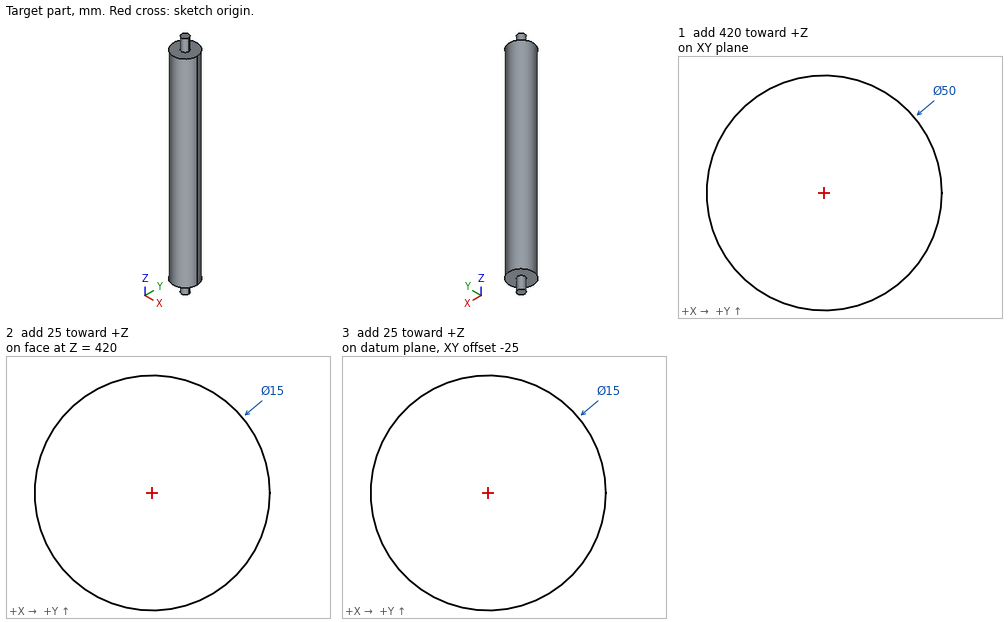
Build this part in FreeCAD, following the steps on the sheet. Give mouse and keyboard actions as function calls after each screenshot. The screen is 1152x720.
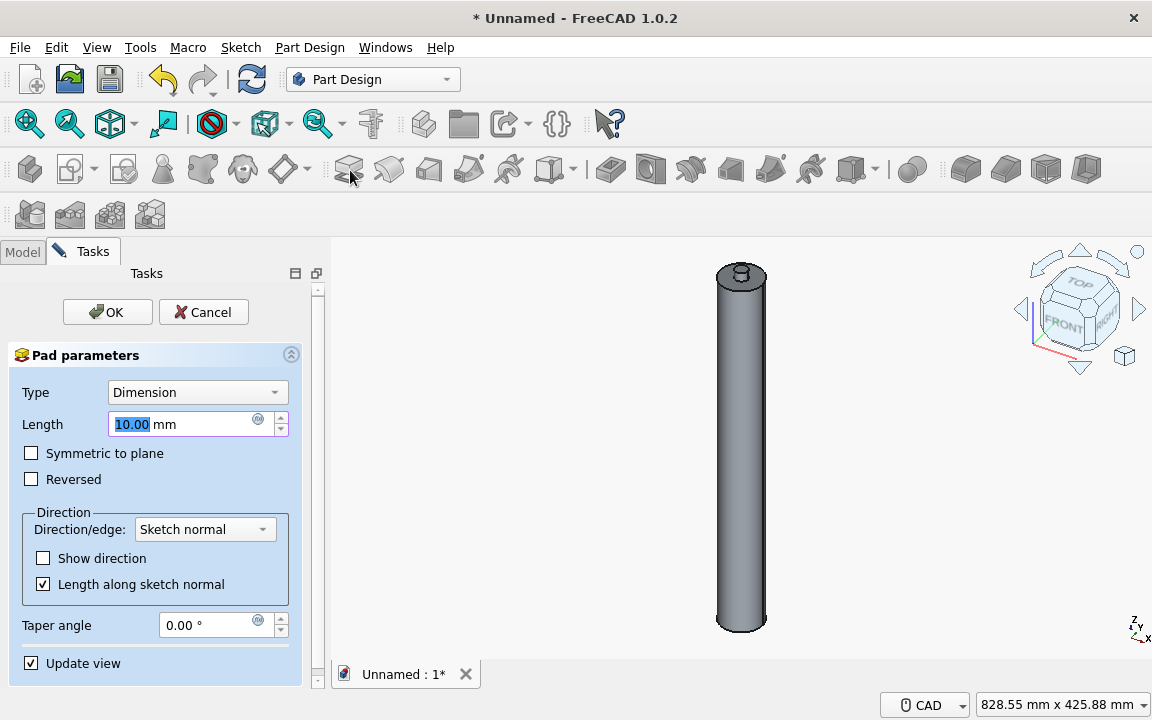
text(25)
key(Tab)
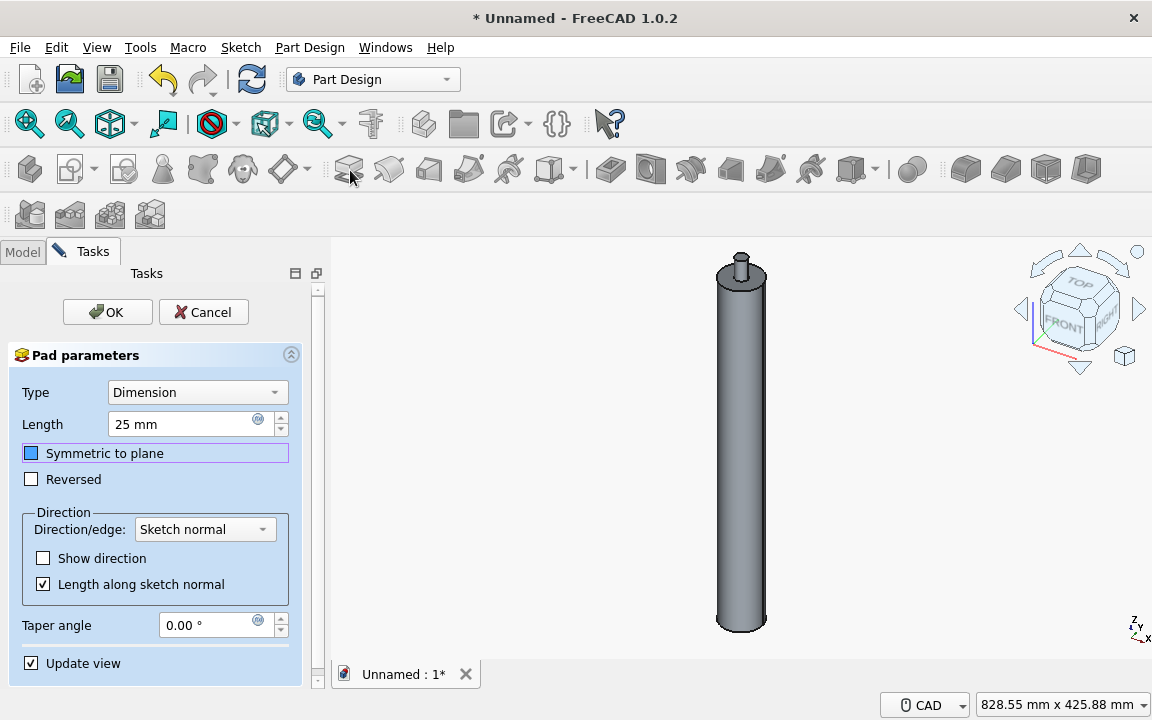
click(108, 312)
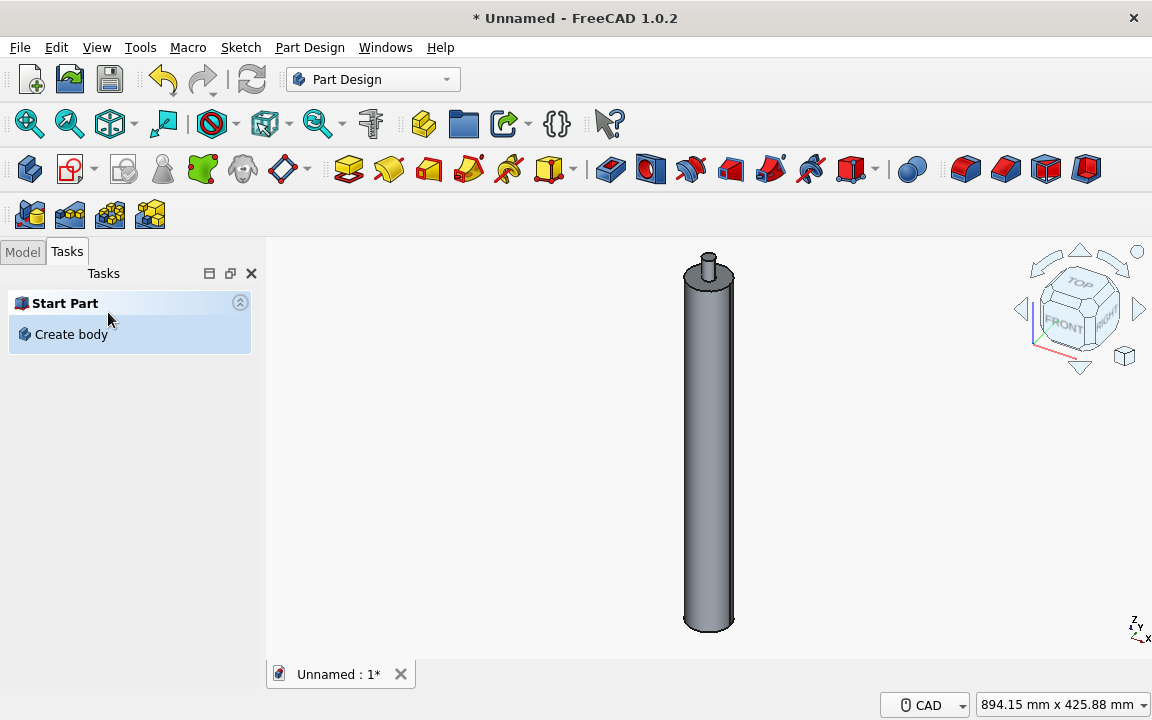
click(23, 251)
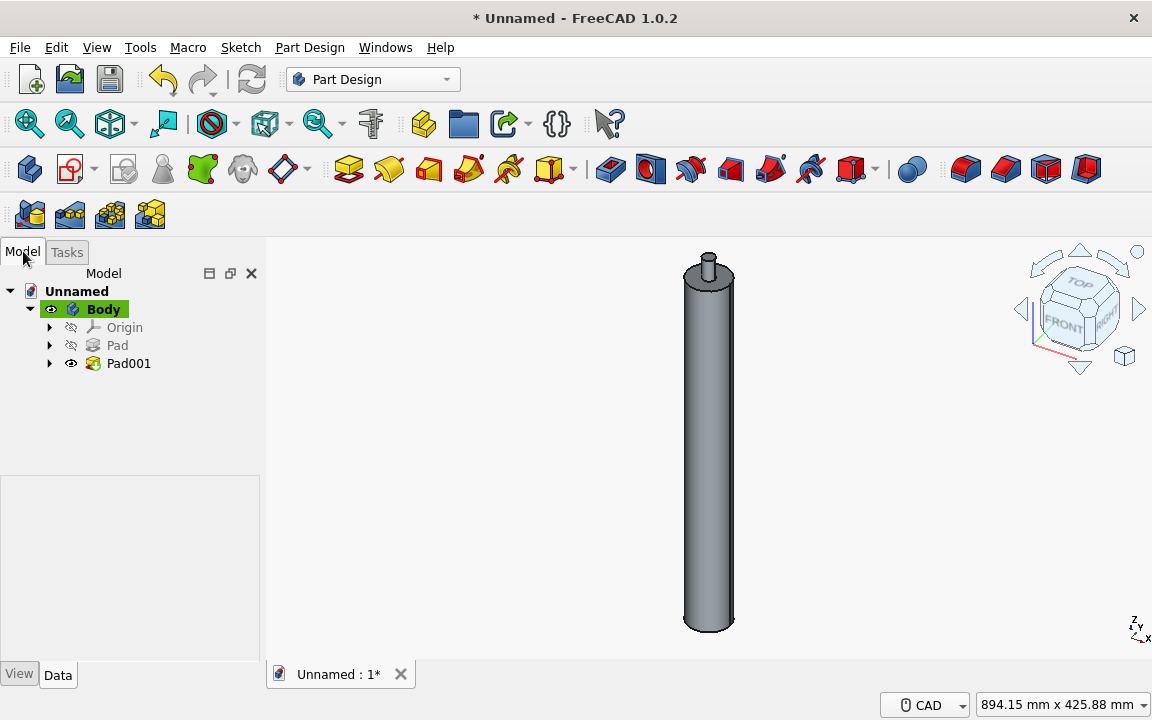
click(50, 327)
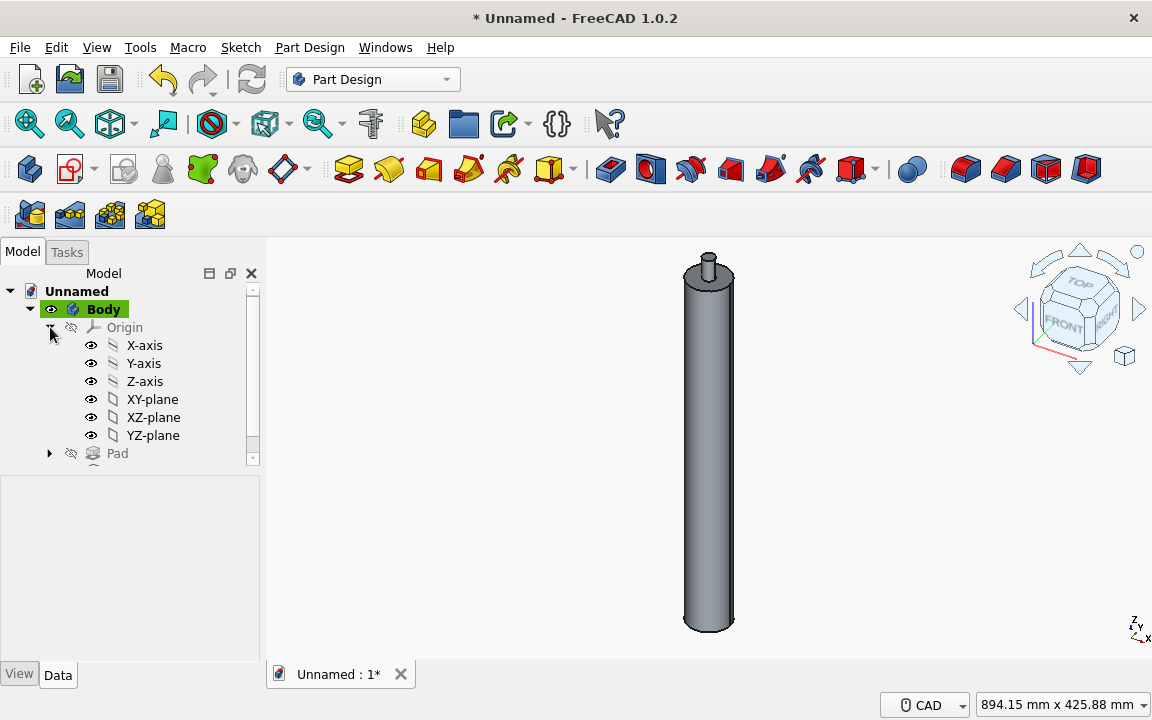
click(136, 399)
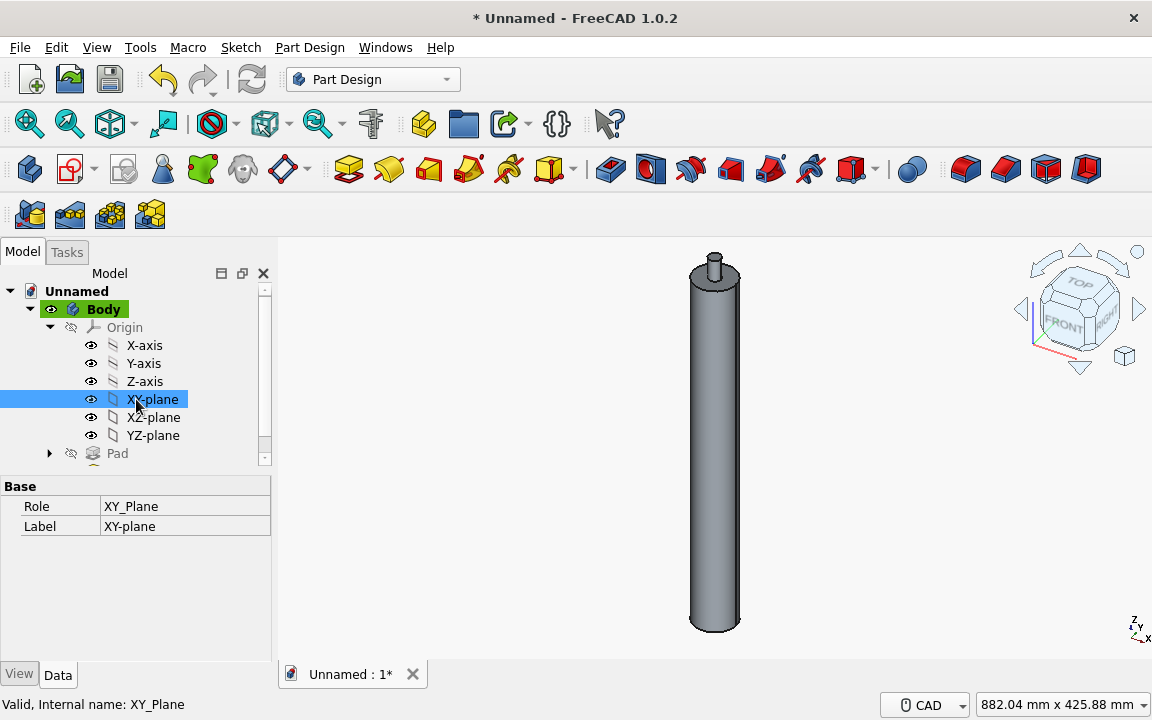
click(284, 170)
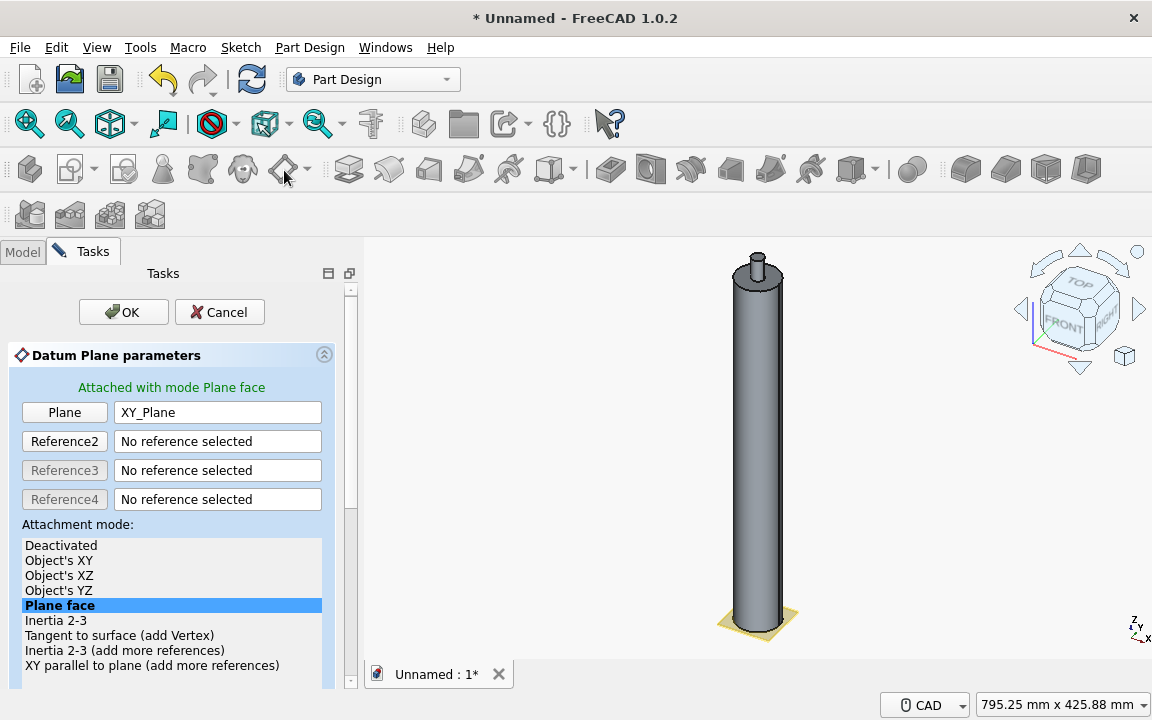
scroll(351, 486, down, 4)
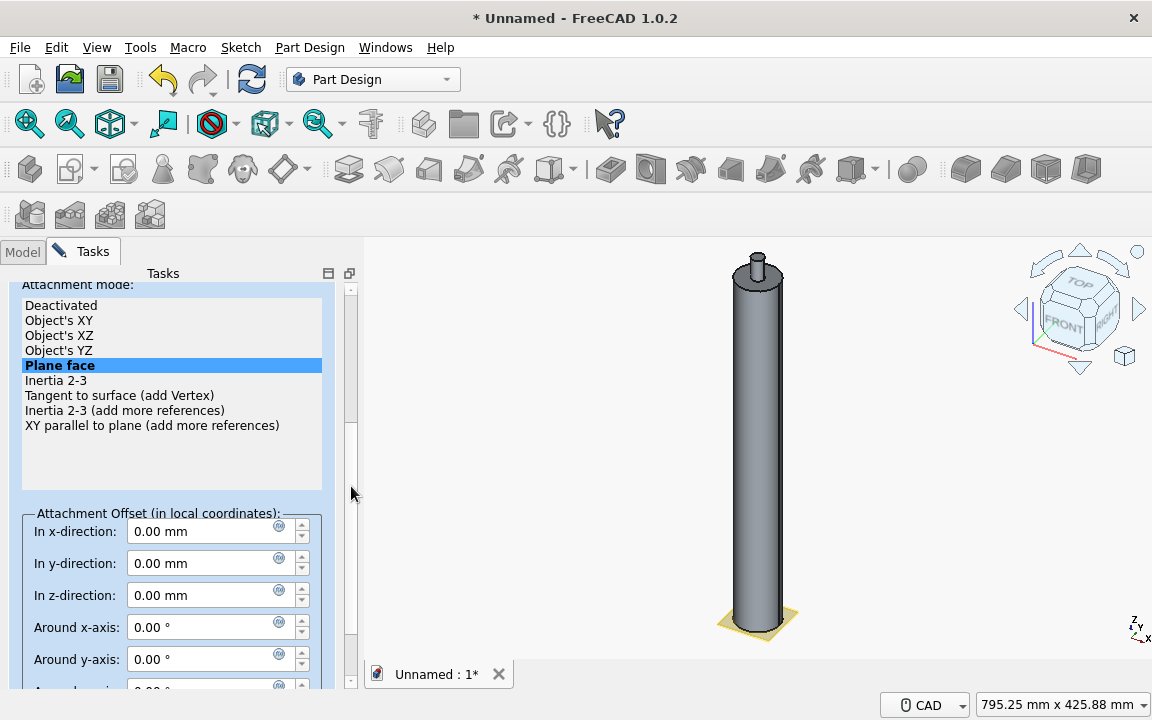
triple_click(210, 595)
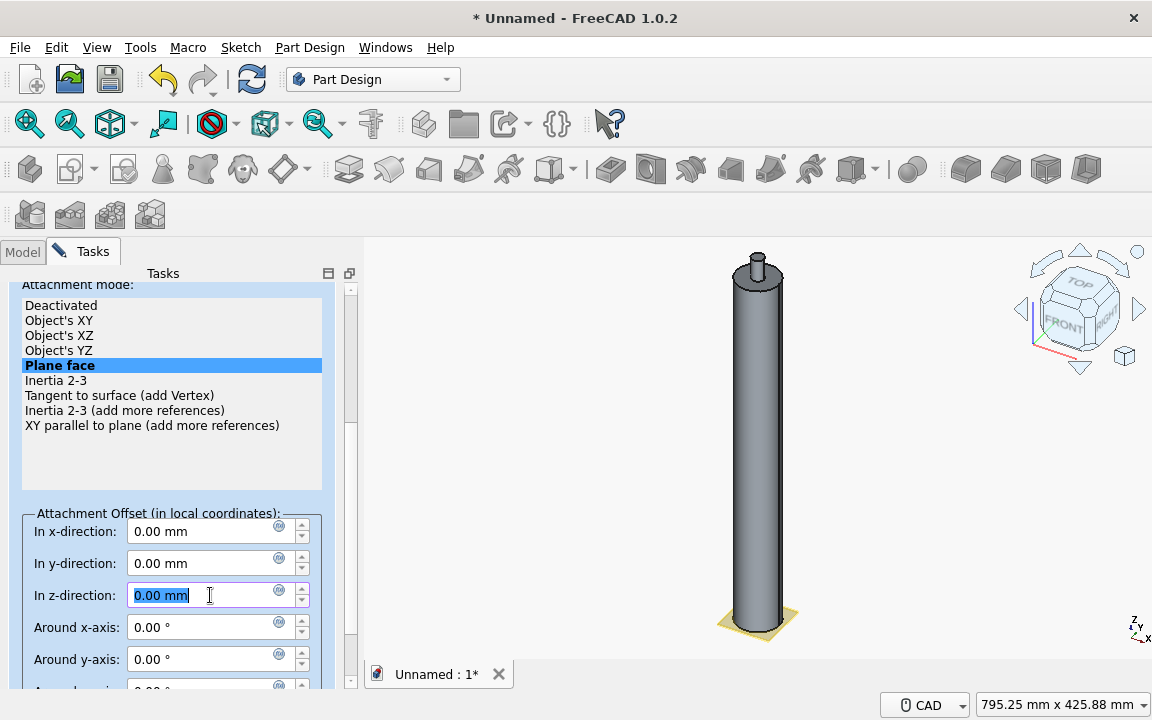
text(-25)
key(Tab)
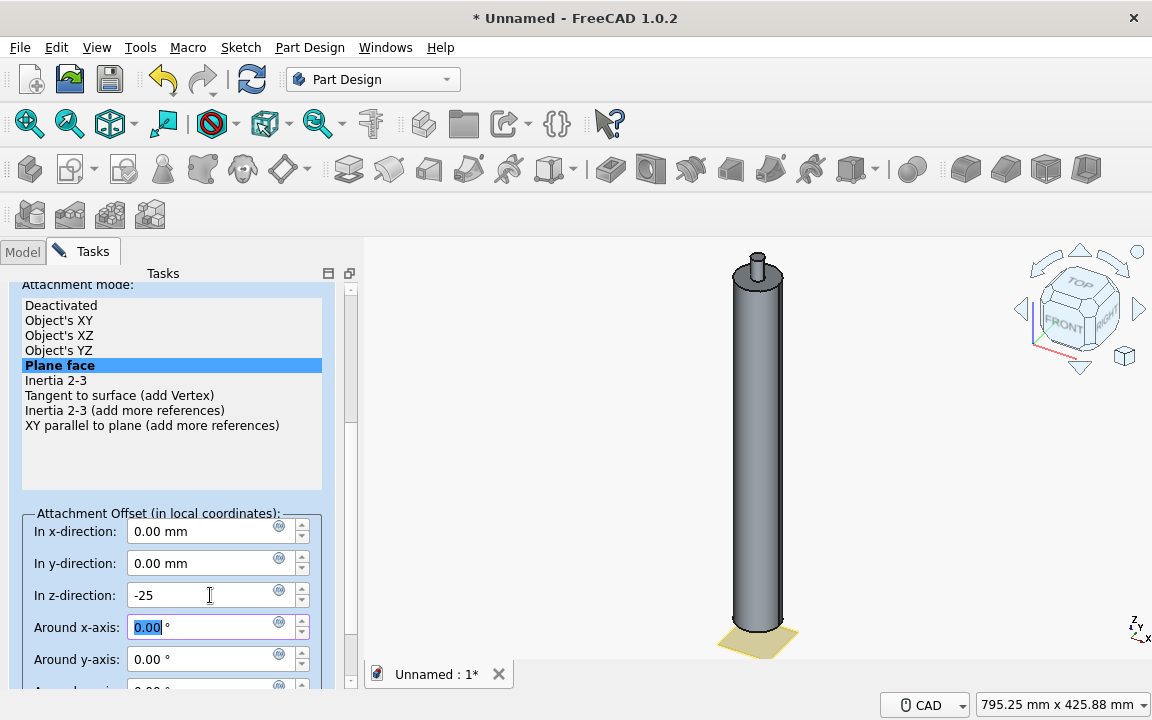
scroll(351, 486, up, 5)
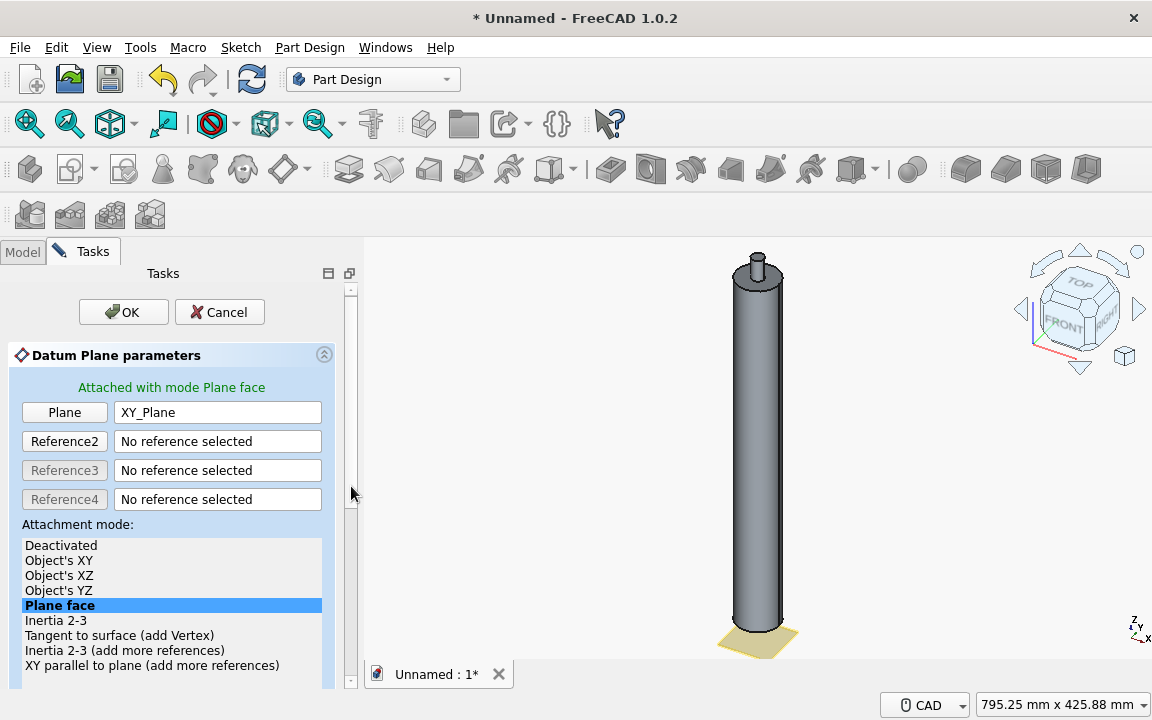
click(124, 312)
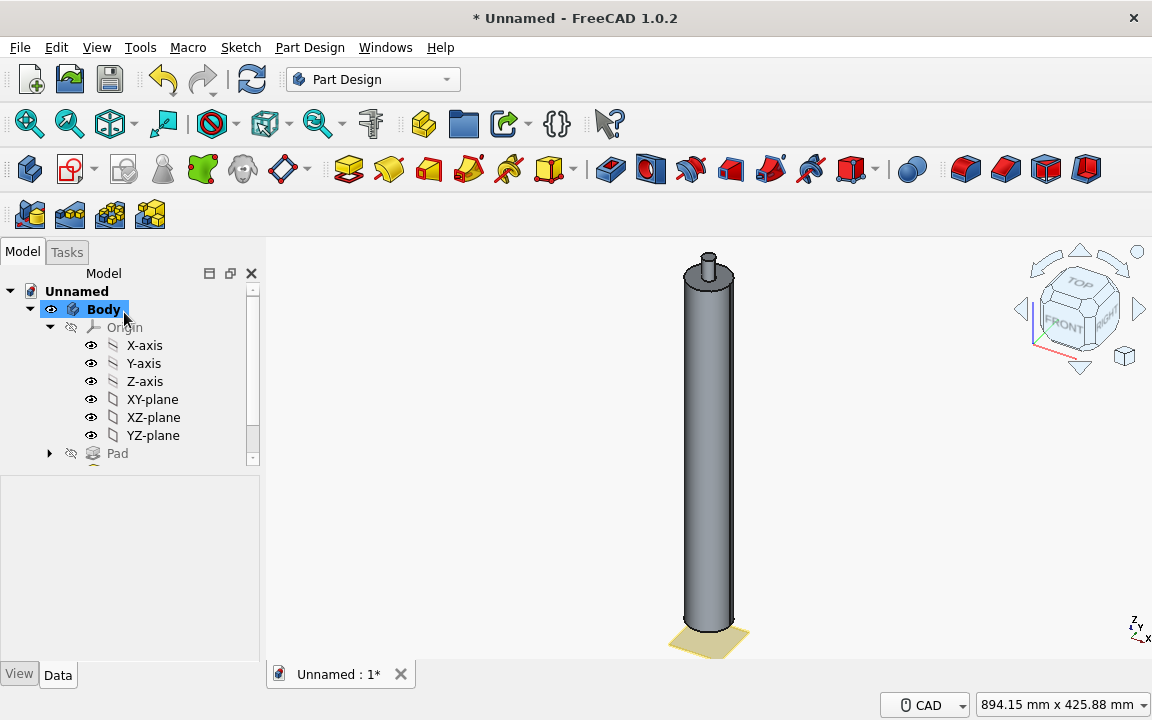
scroll(100, 377, down, 3)